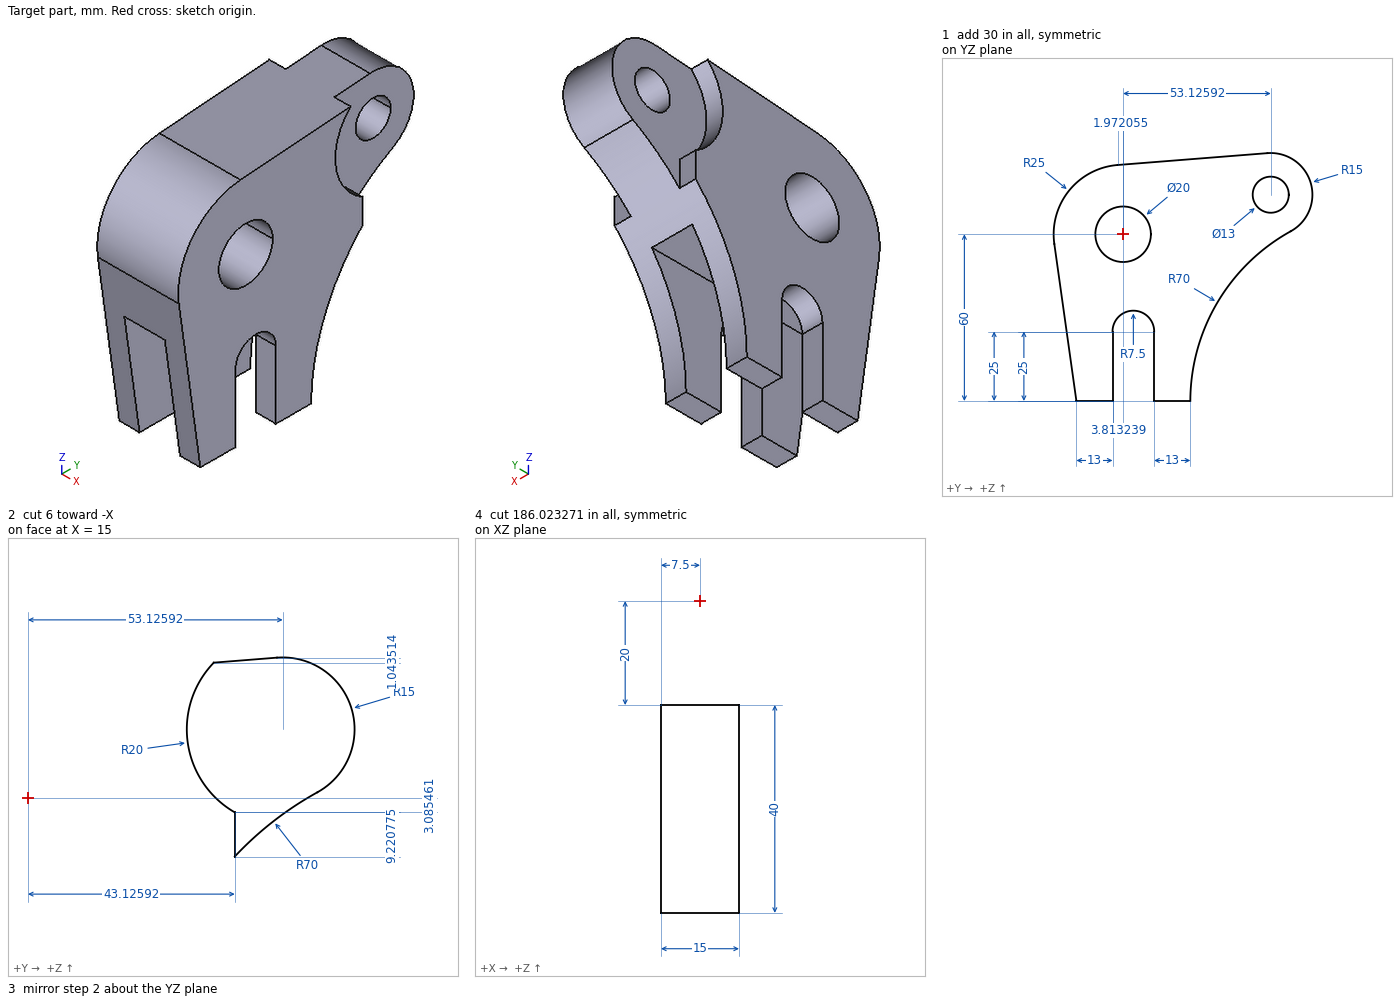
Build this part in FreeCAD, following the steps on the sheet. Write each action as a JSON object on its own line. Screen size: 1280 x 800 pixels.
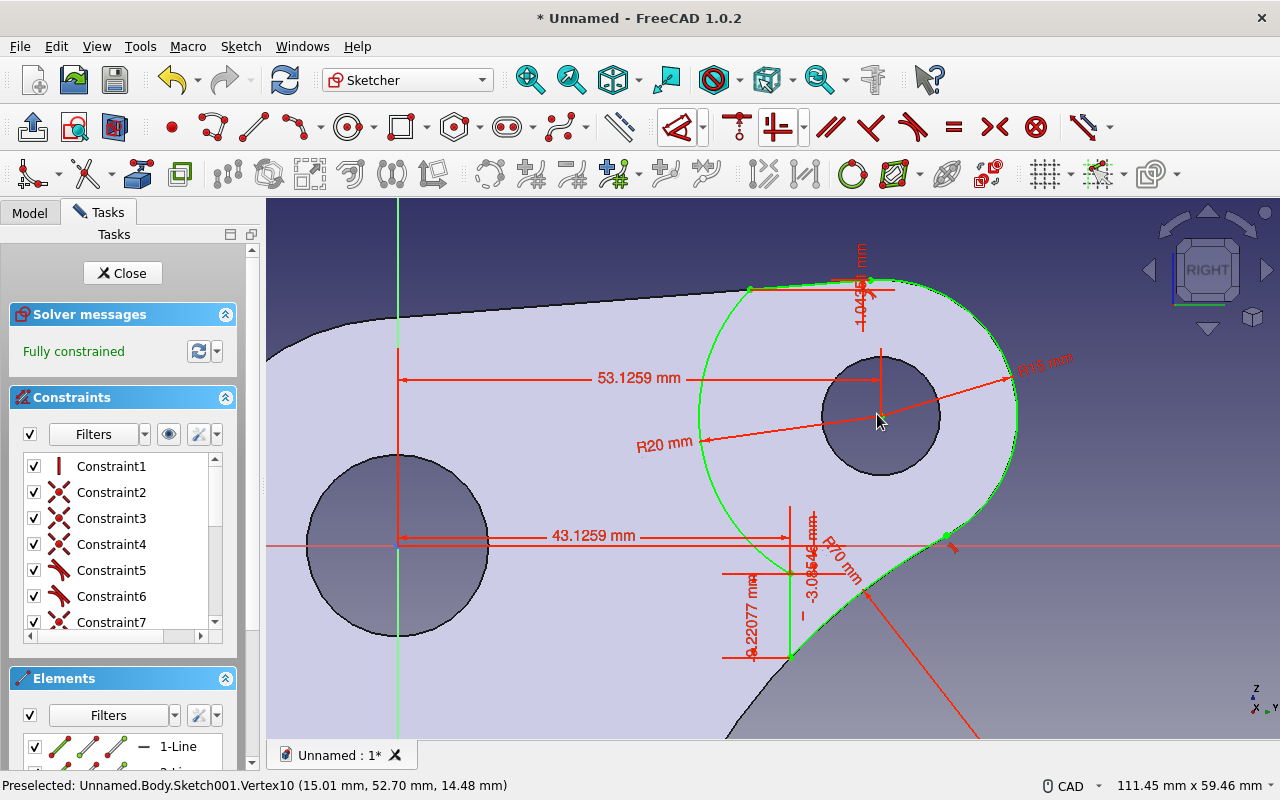
{"action": "left_click", "coordinate": [123, 273]}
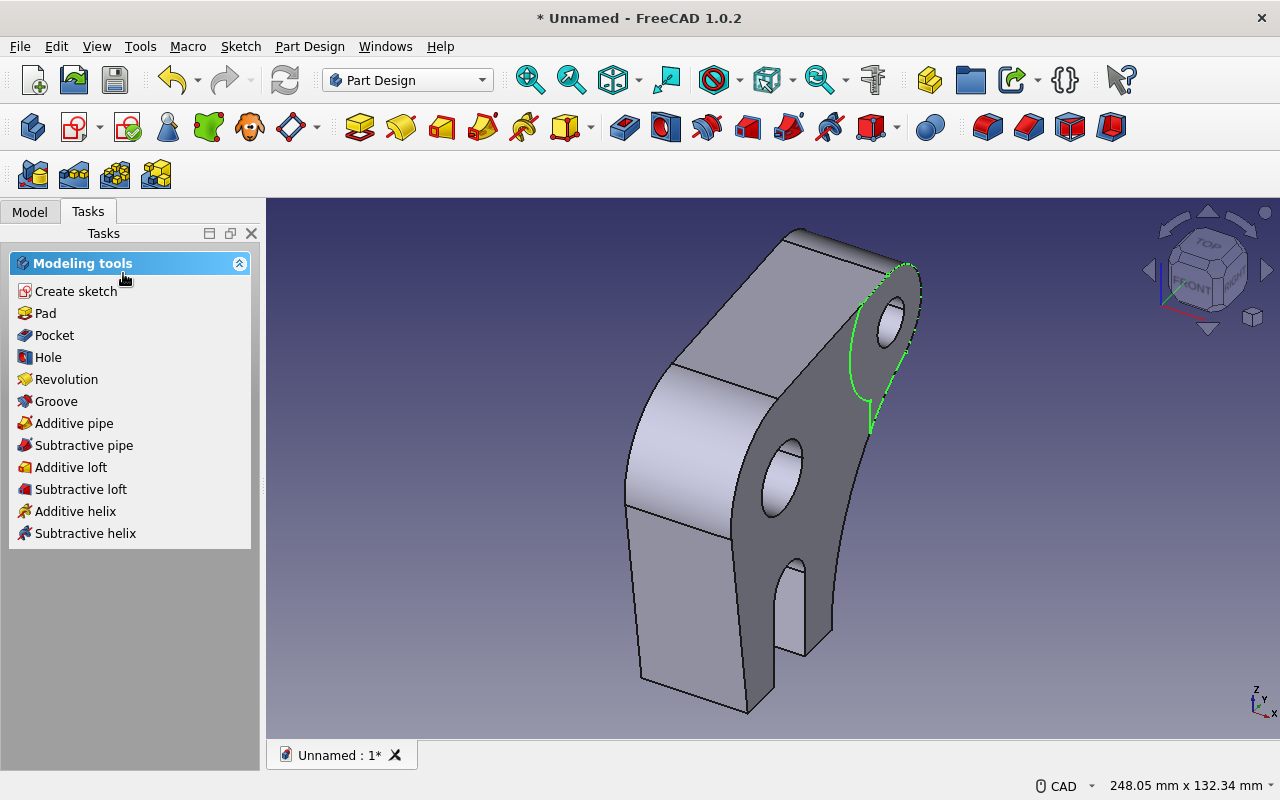
{"action": "left_click", "coordinate": [625, 128]}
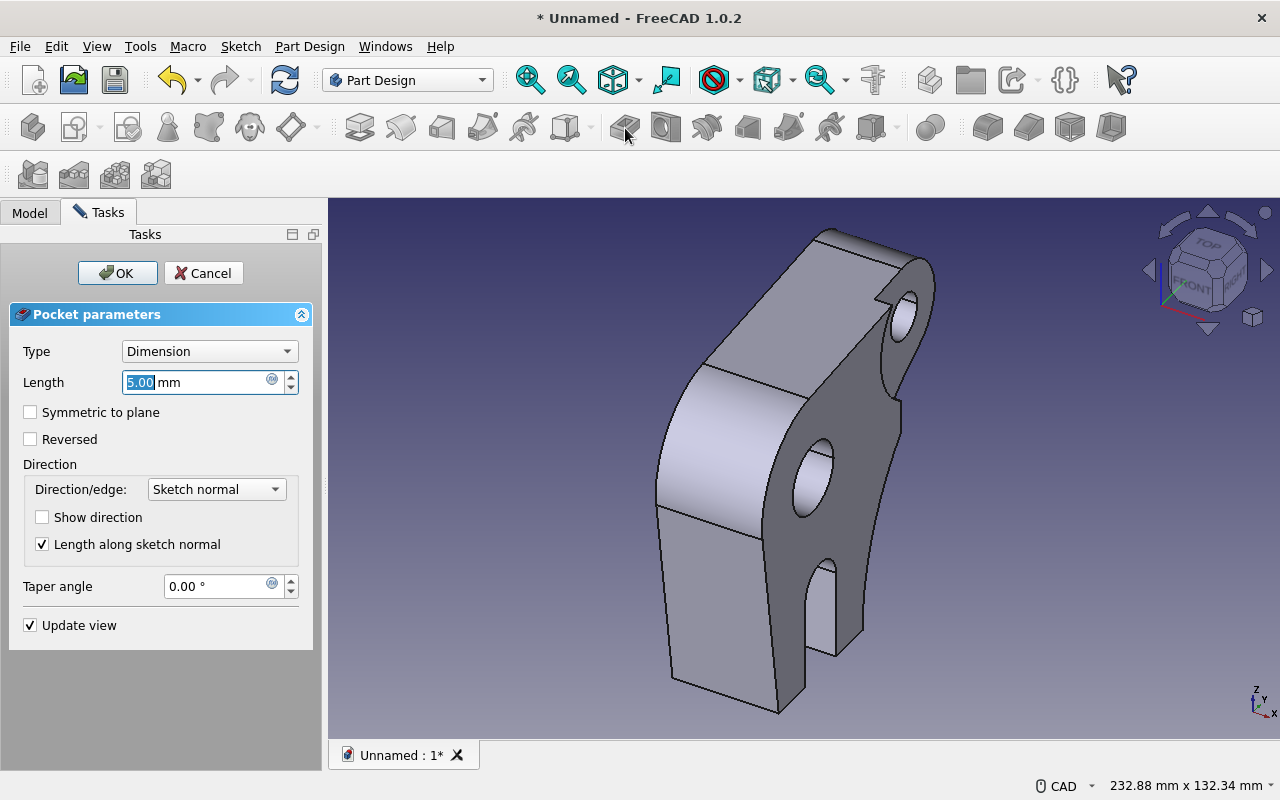
{"action": "type", "text": "6"}
{"action": "key", "text": "Tab"}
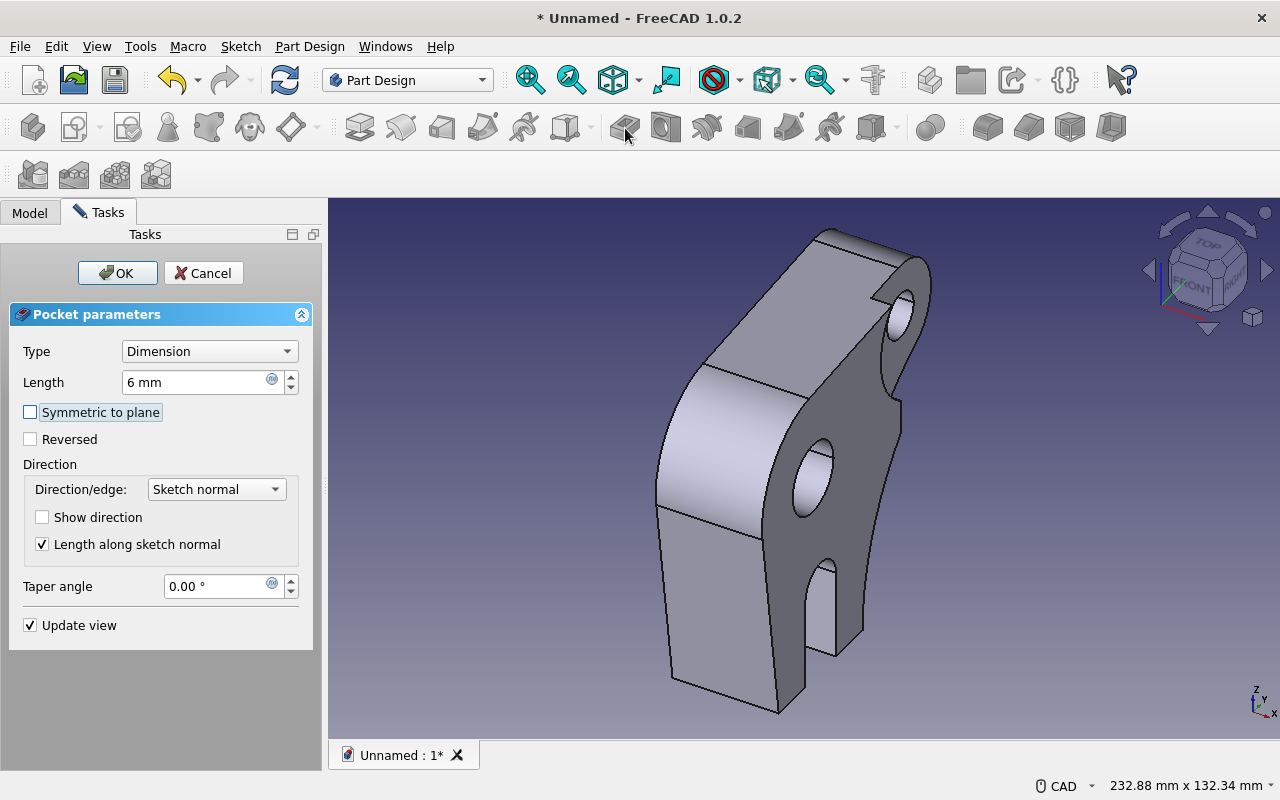
{"action": "left_click", "coordinate": [118, 273]}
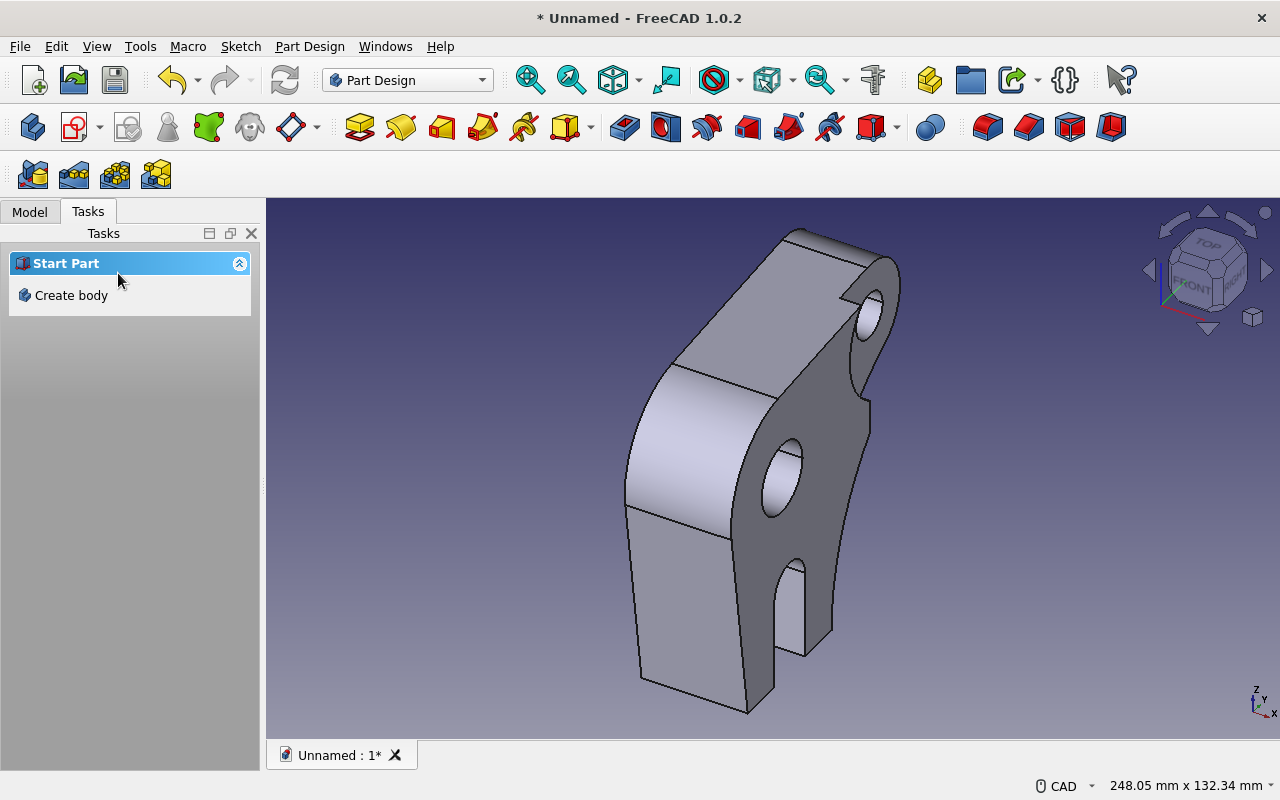
{"action": "left_click", "coordinate": [30, 212]}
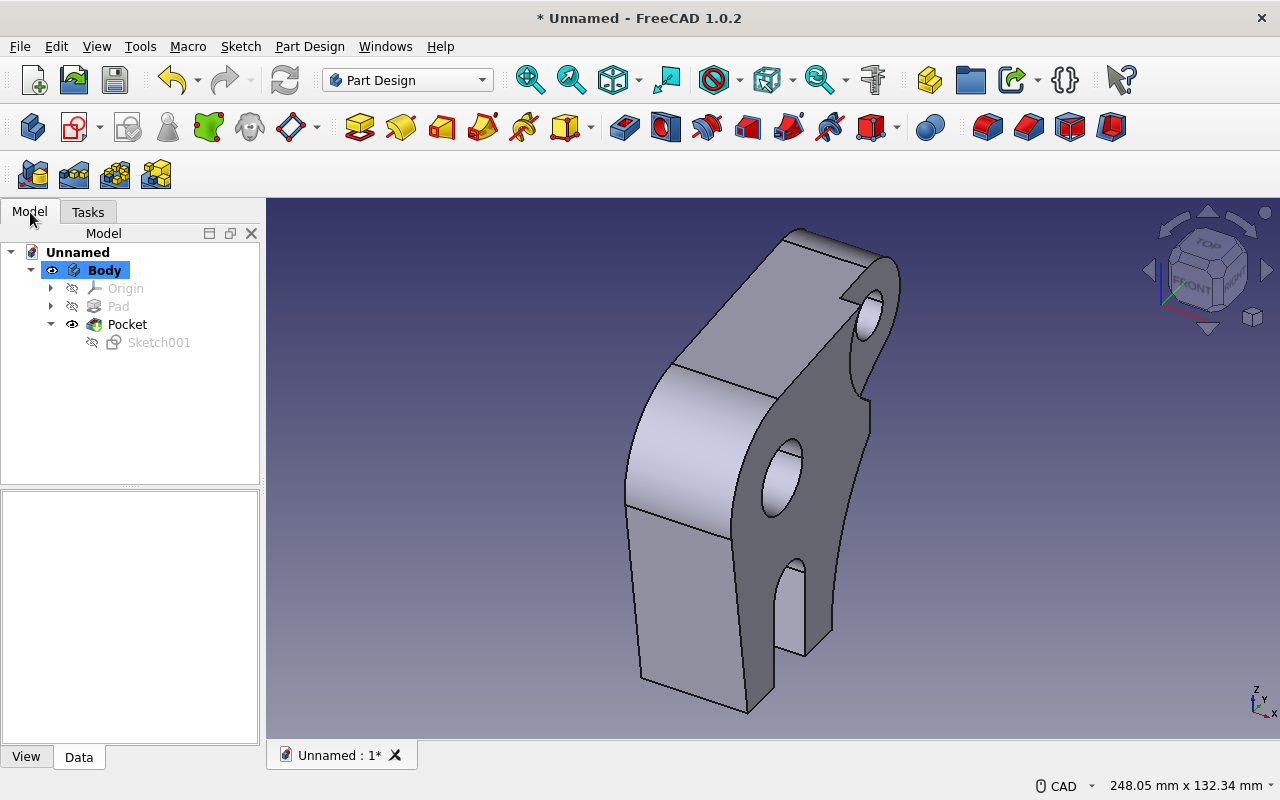
{"action": "left_click", "coordinate": [117, 324]}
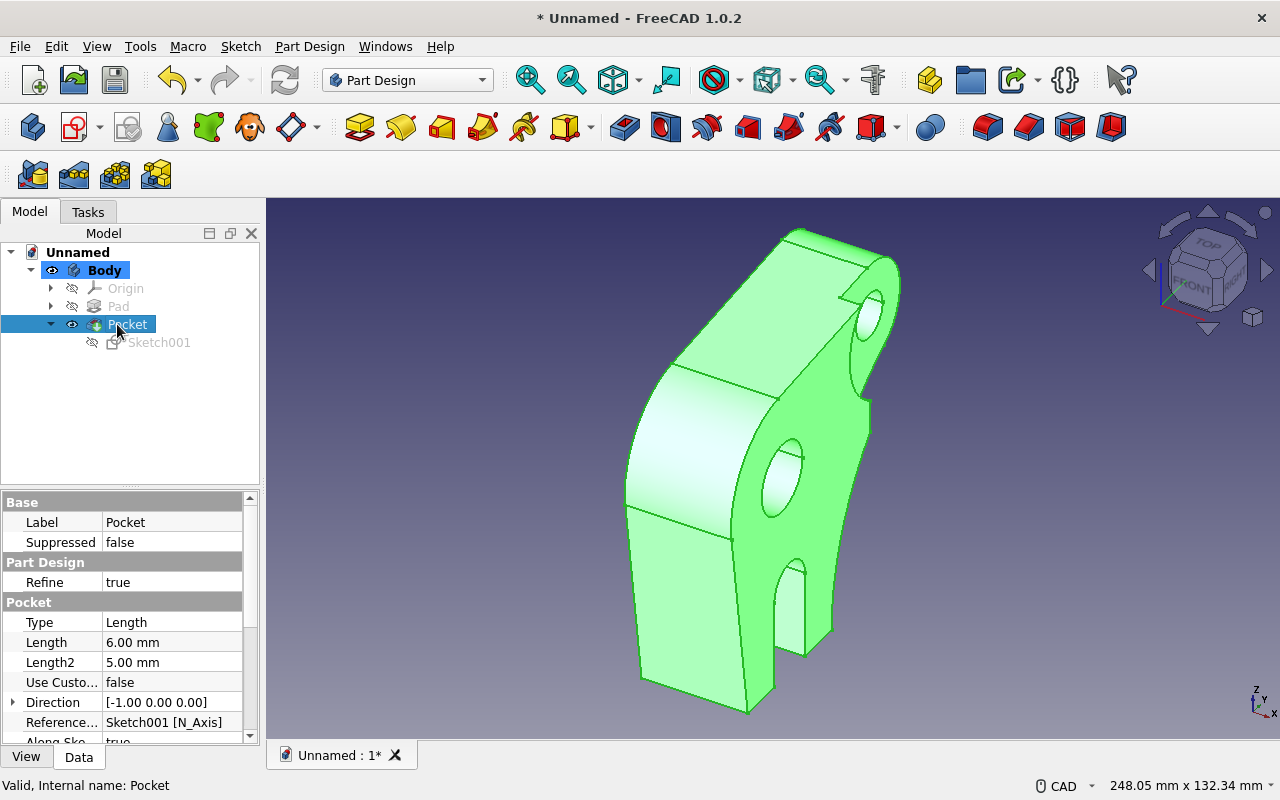
{"action": "left_click", "coordinate": [33, 174]}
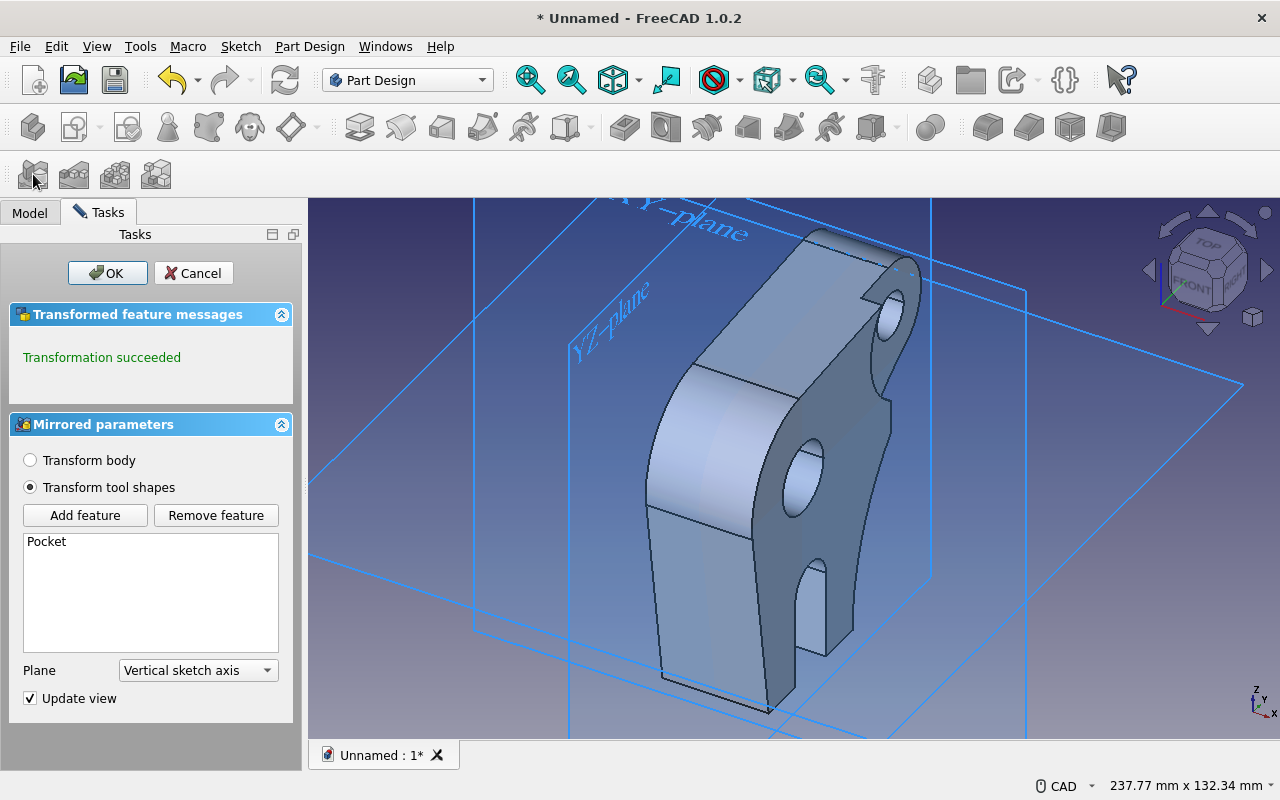
{"action": "left_click", "coordinate": [199, 670]}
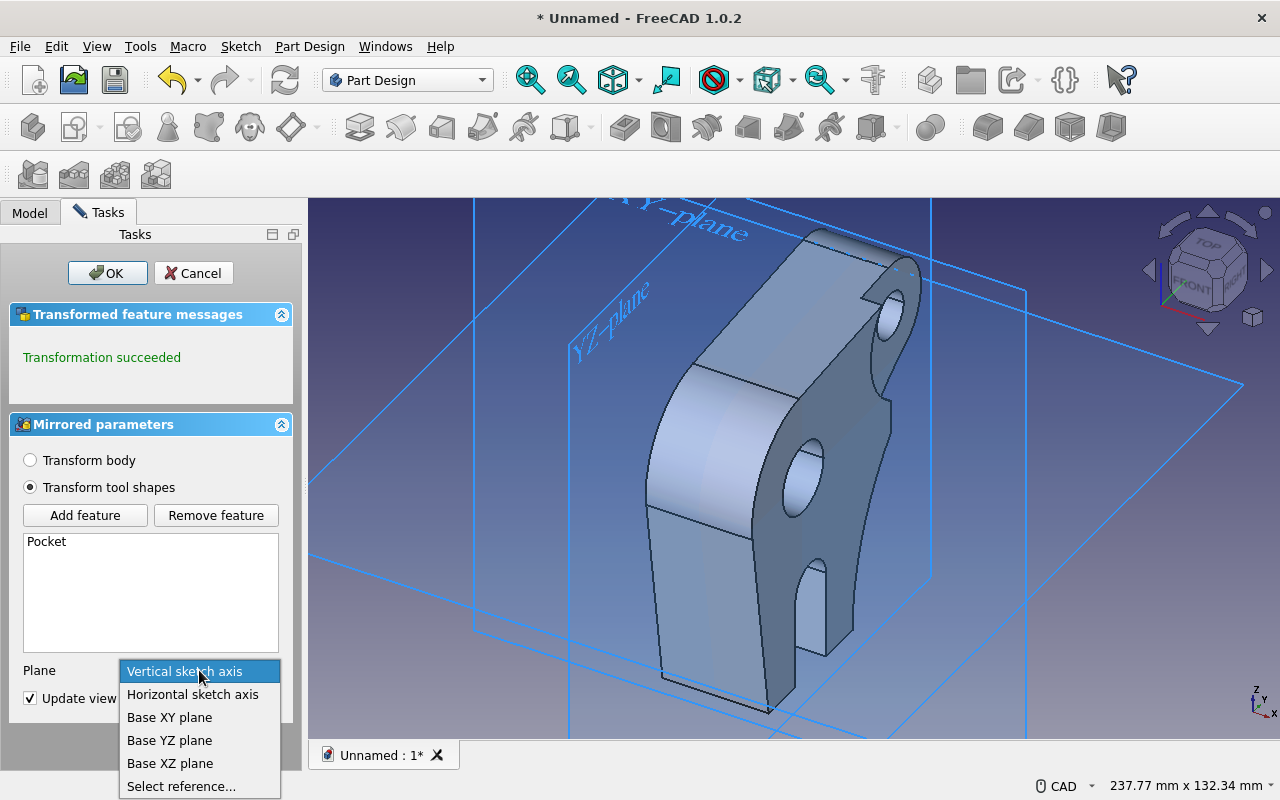
{"action": "left_click", "coordinate": [198, 740]}